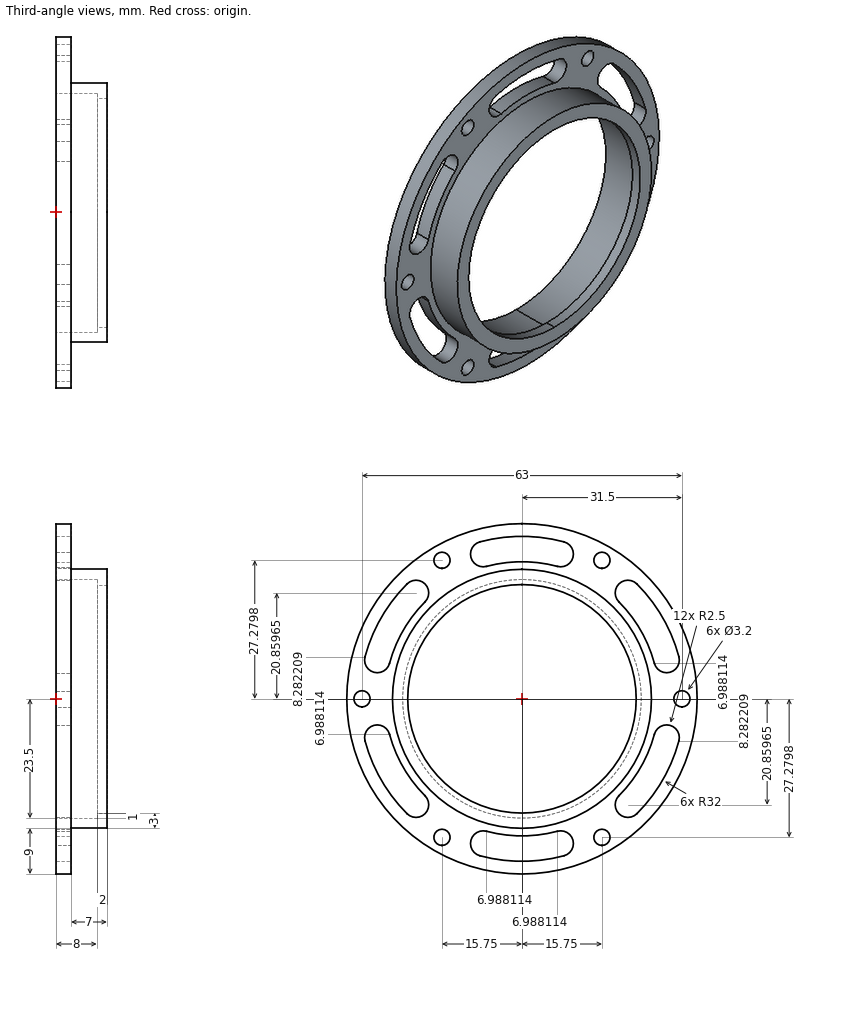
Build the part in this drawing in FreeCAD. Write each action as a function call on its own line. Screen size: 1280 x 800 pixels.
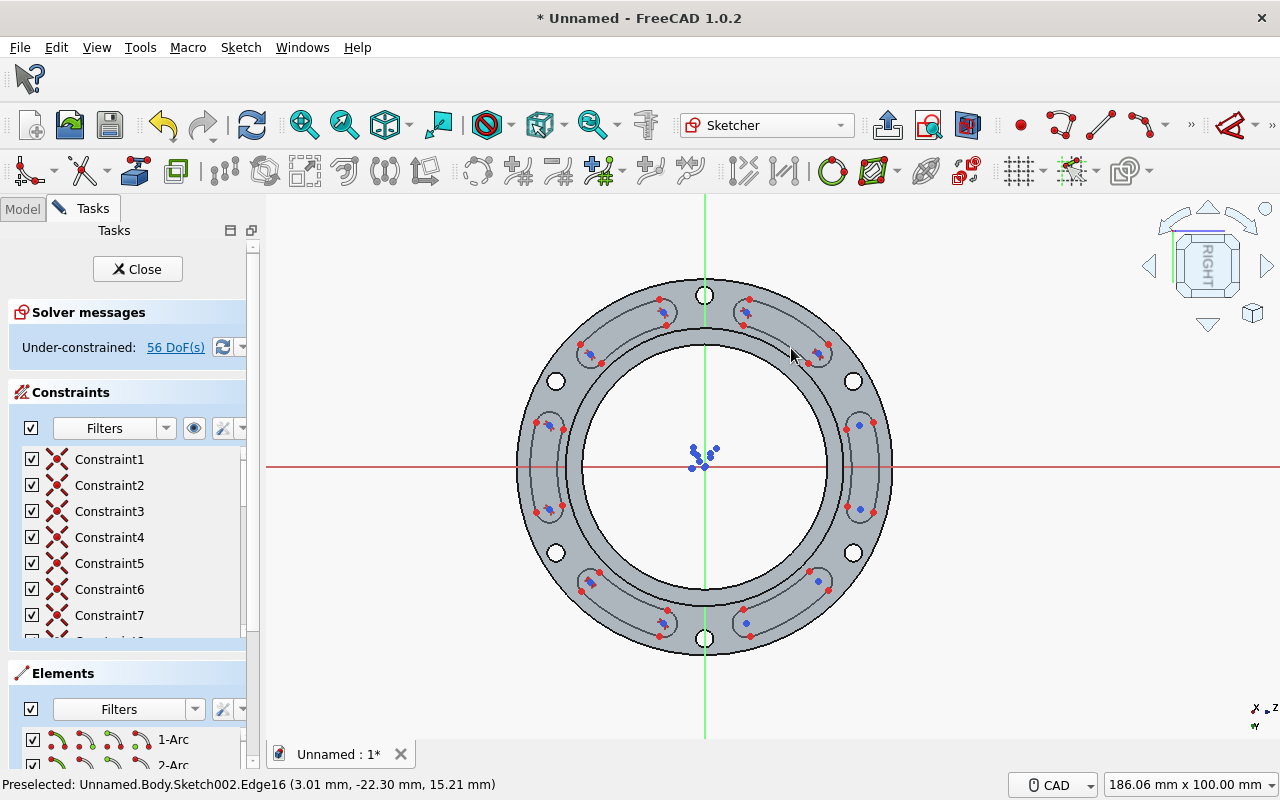
click(851, 484)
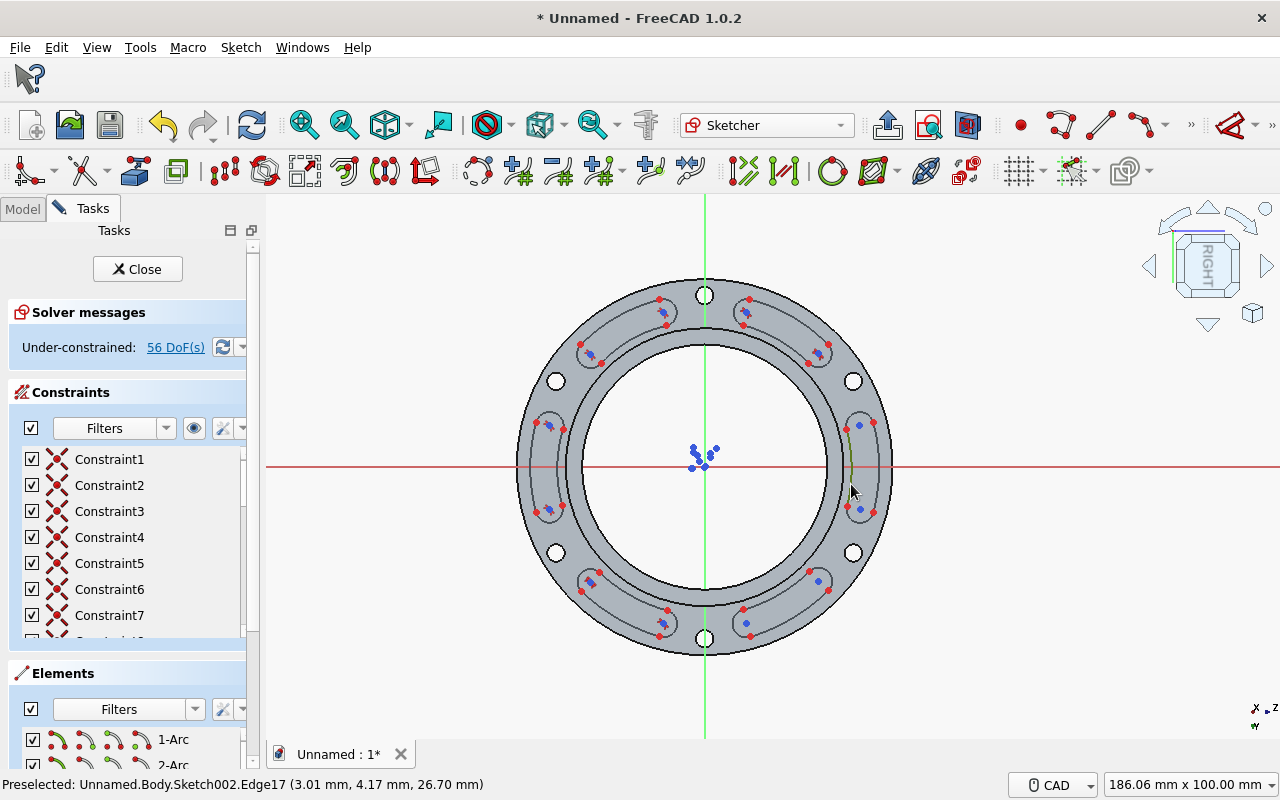
click(850, 518)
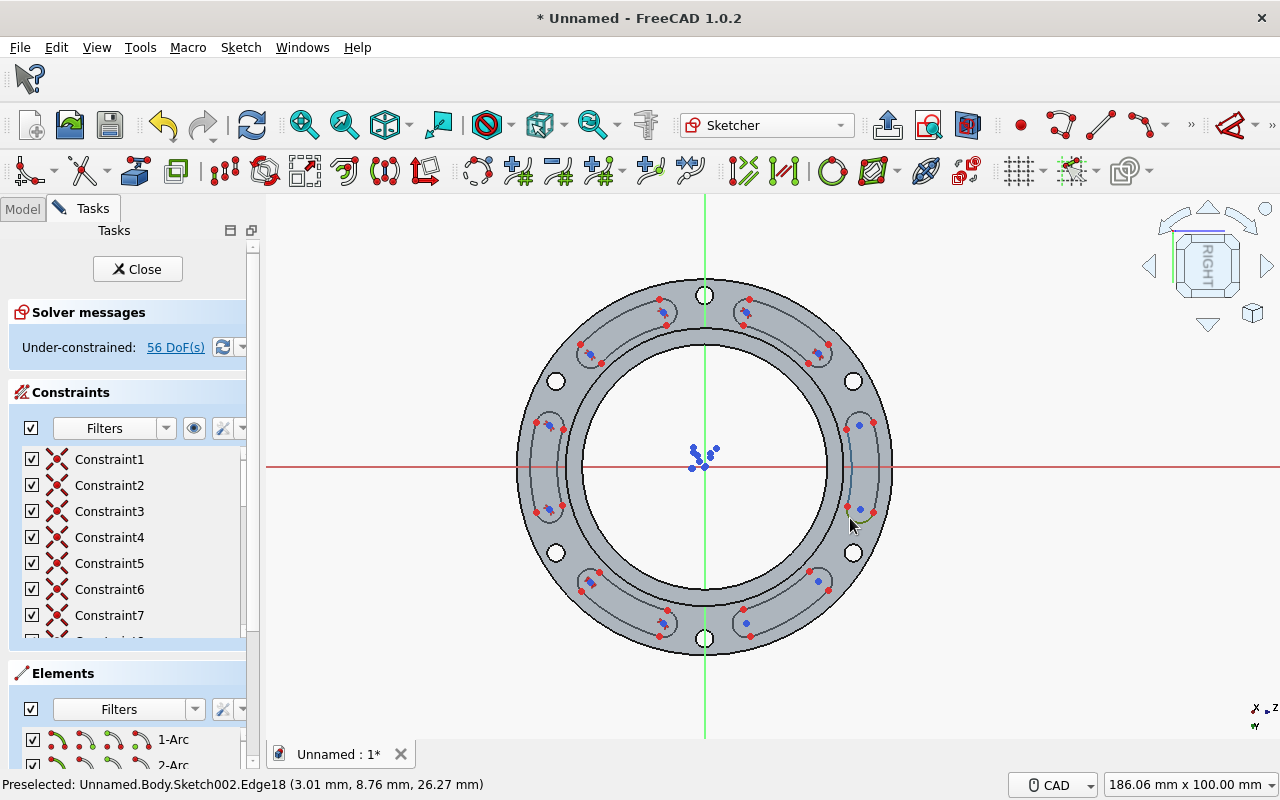
key(t)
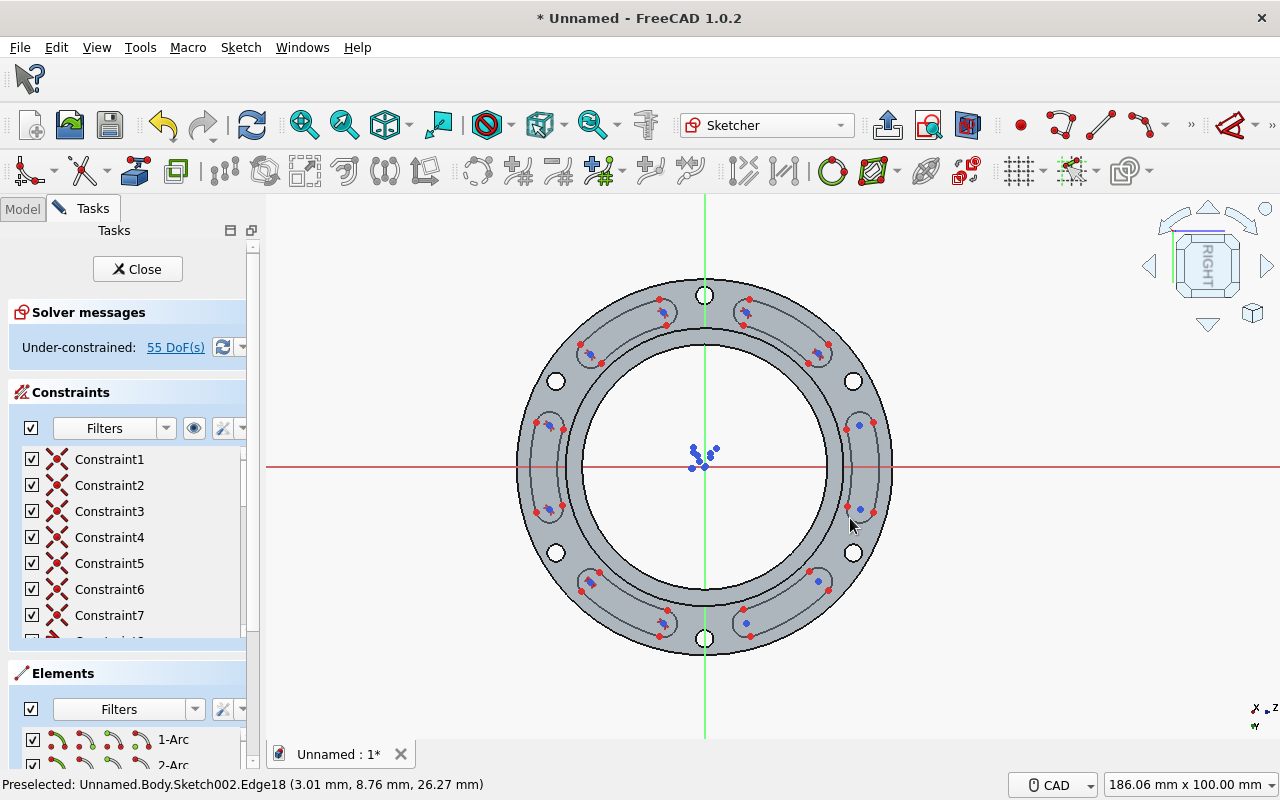
click(851, 483)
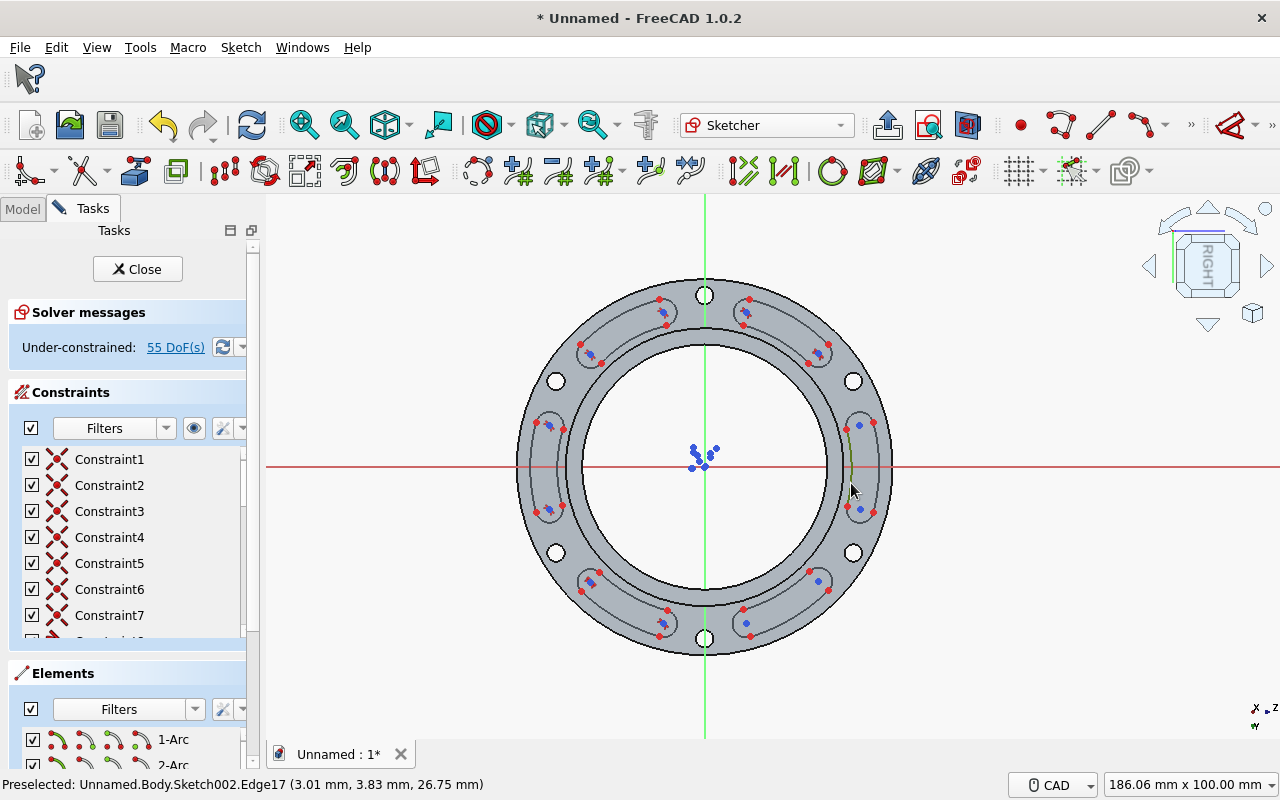
click(865, 413)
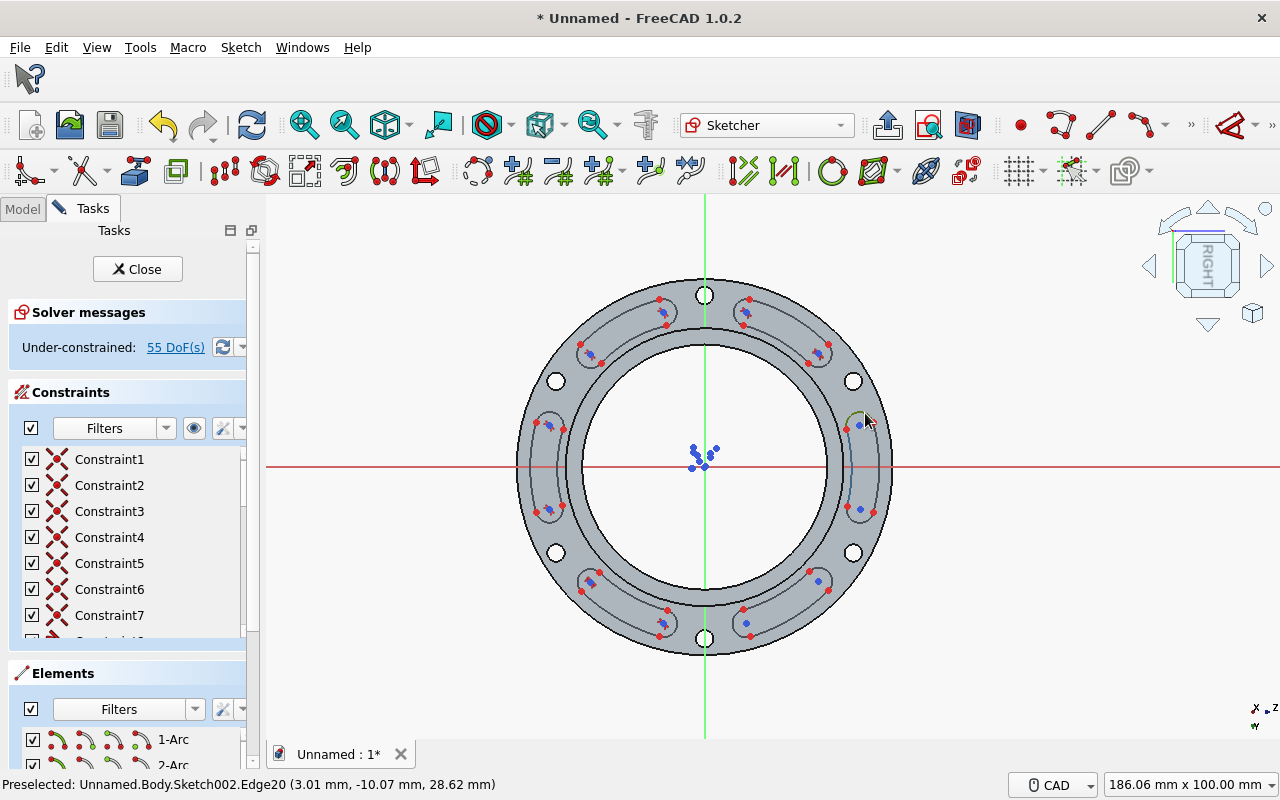
key(t)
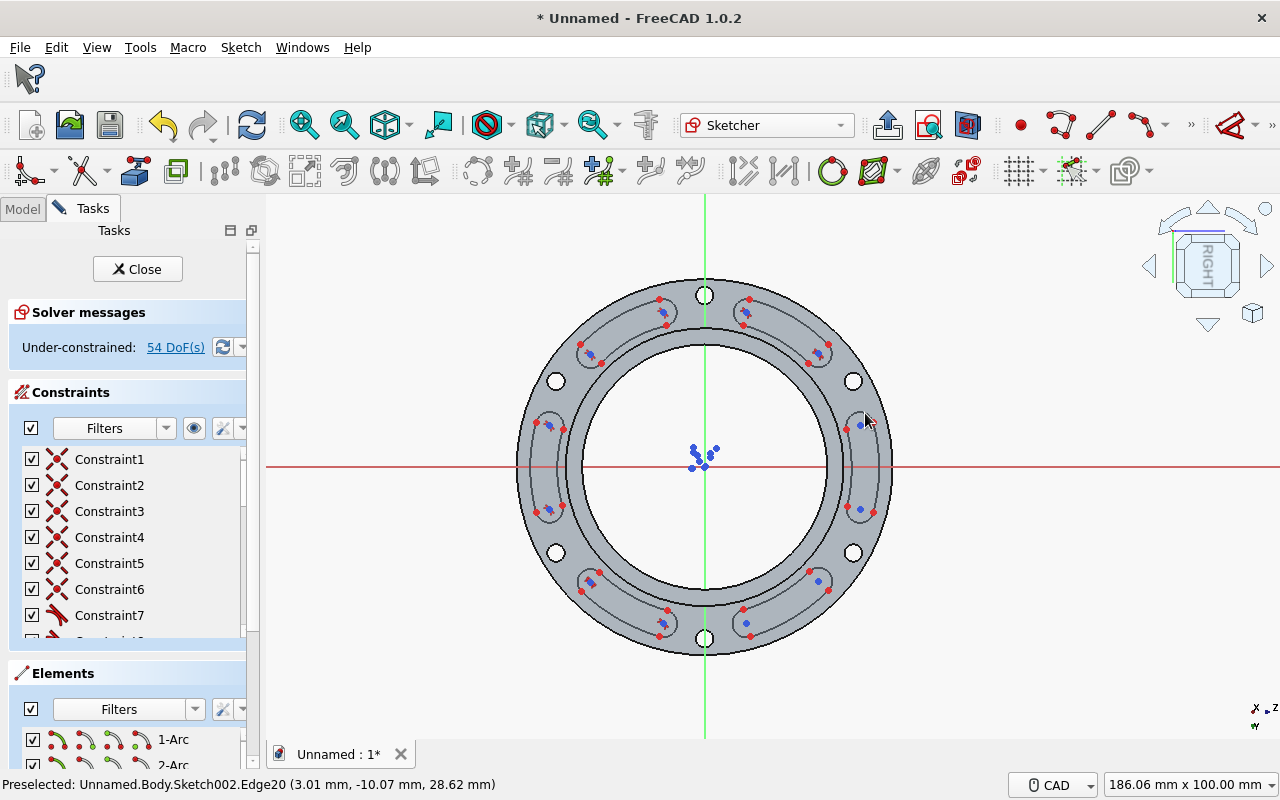
click(850, 518)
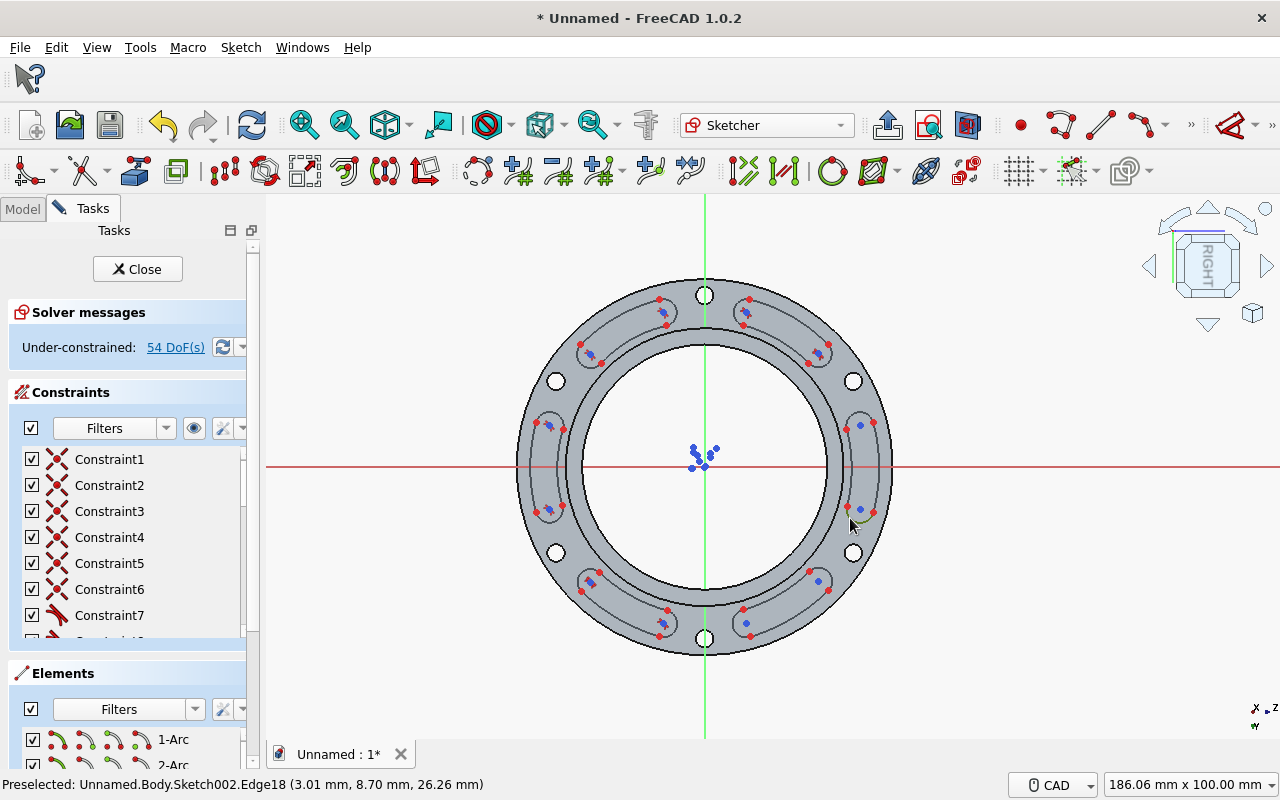
click(878, 486)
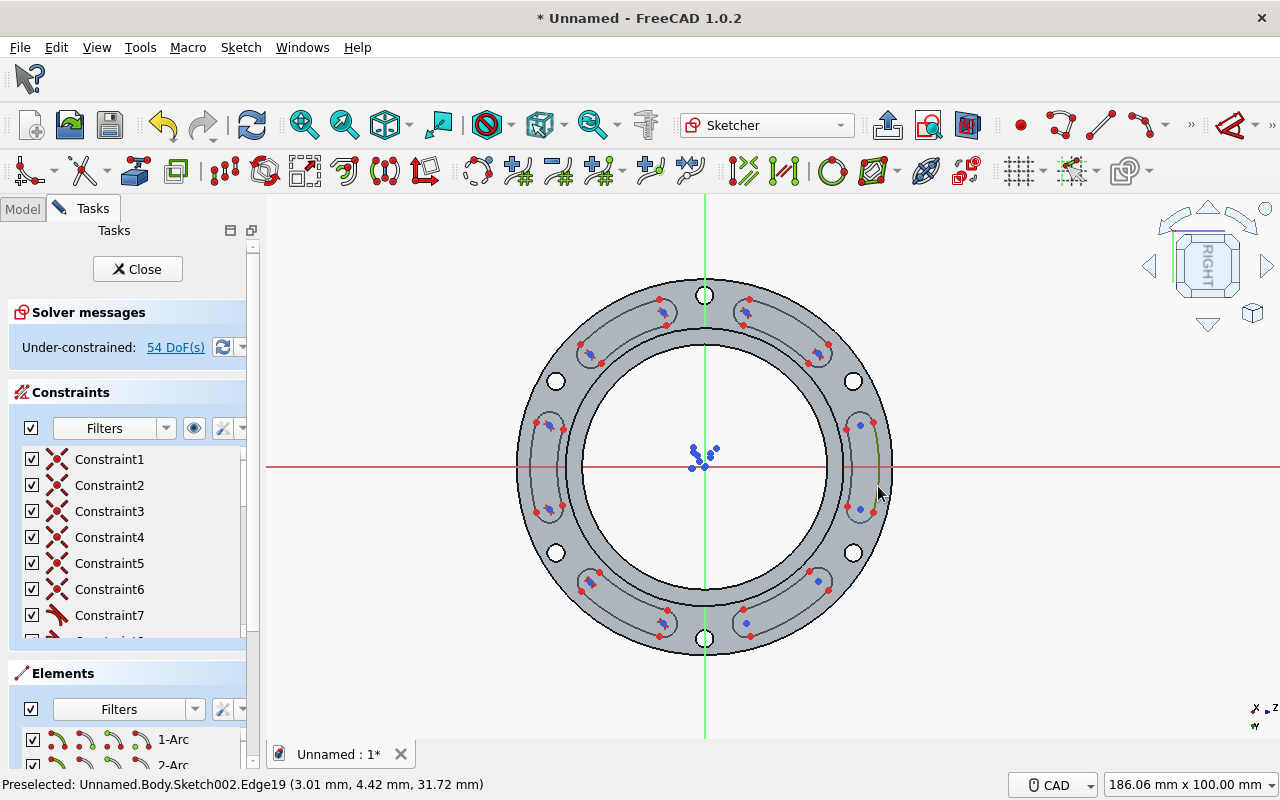
key(t)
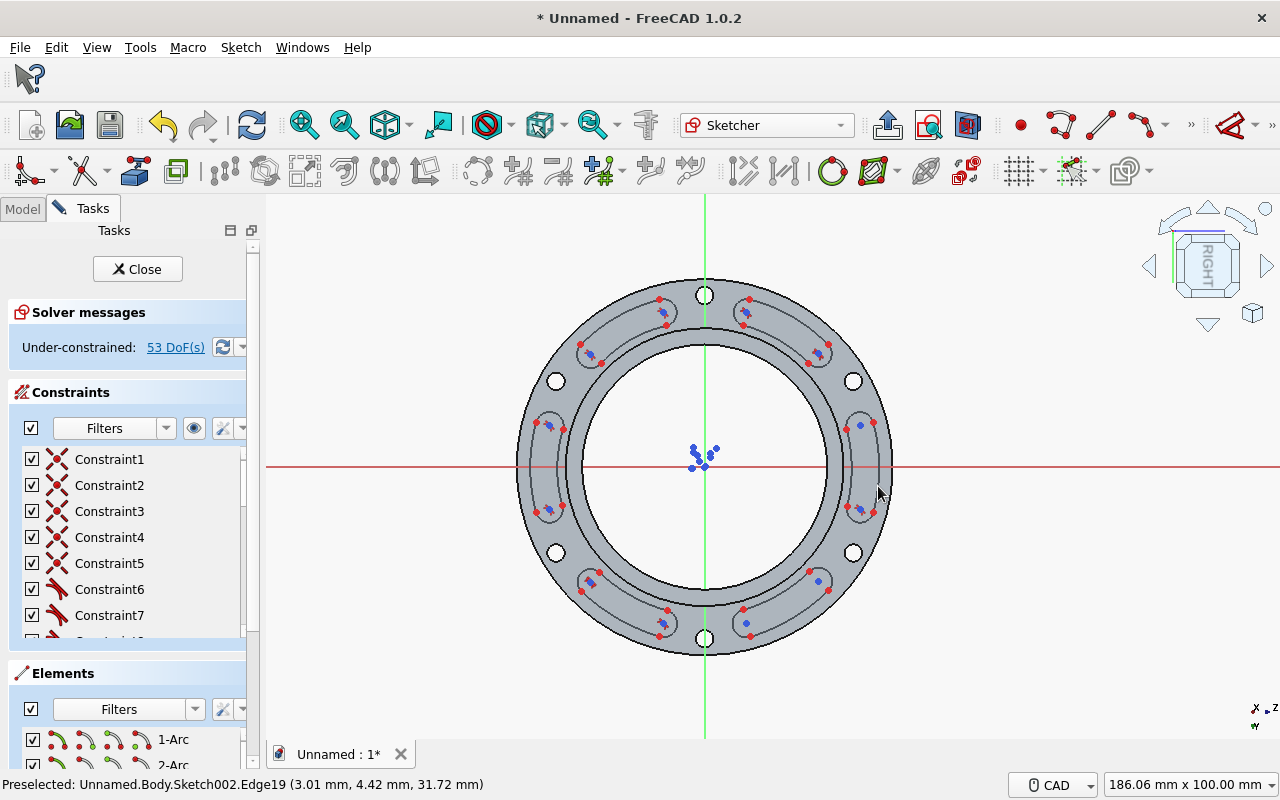
click(878, 486)